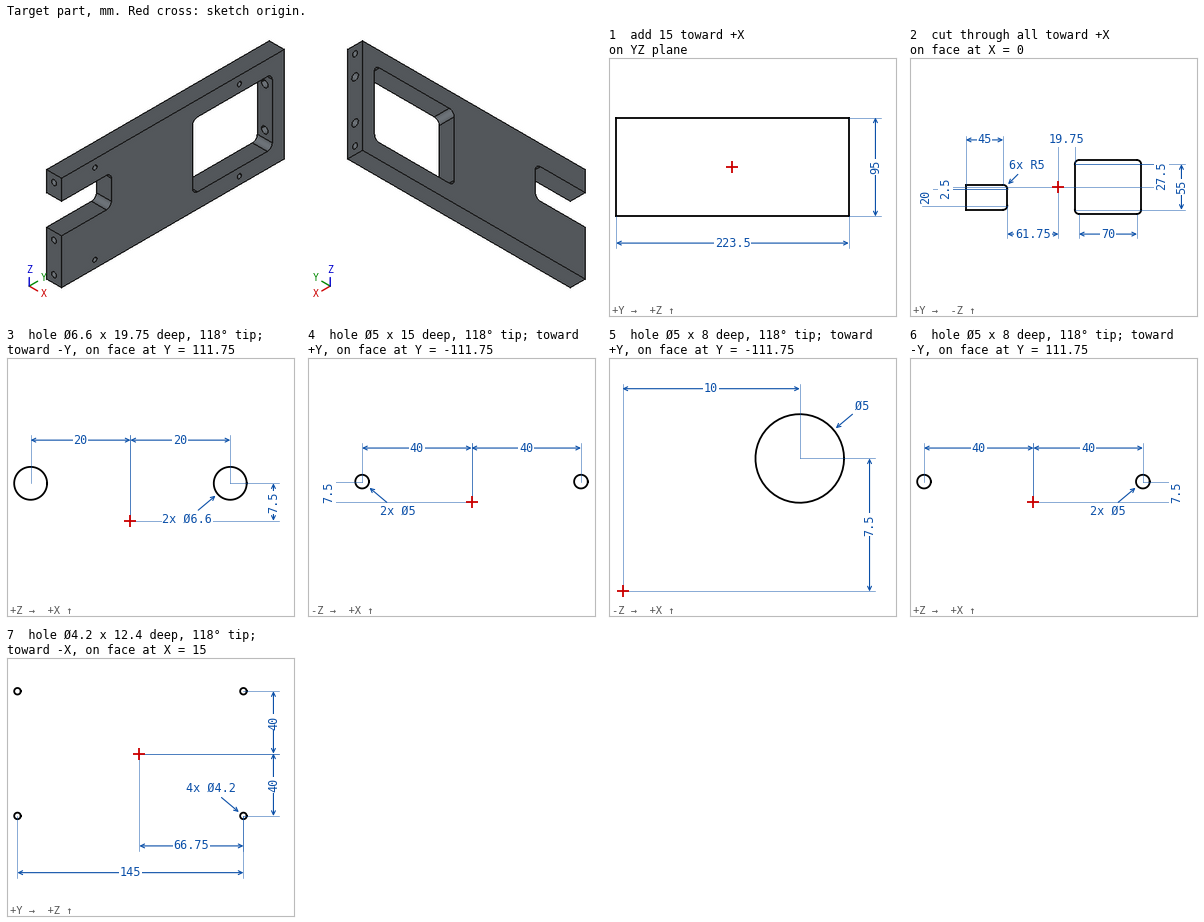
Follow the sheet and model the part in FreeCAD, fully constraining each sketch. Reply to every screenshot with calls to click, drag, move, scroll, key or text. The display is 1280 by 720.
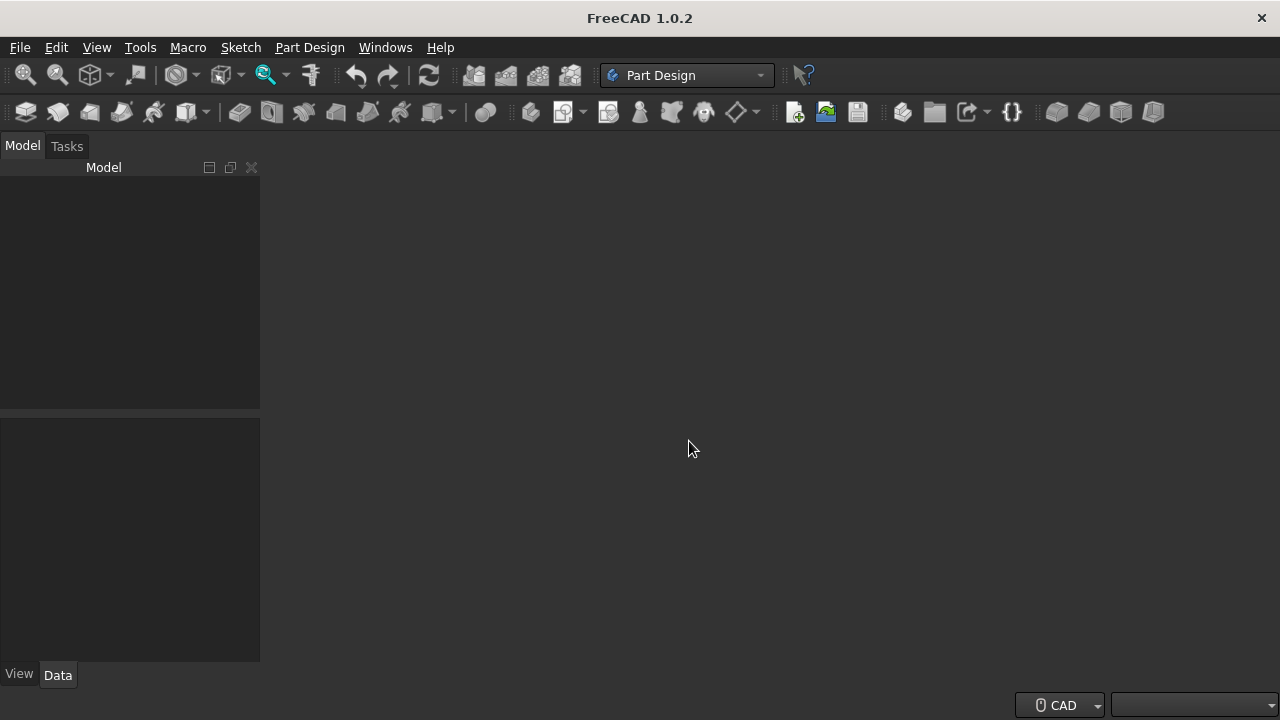
click(794, 112)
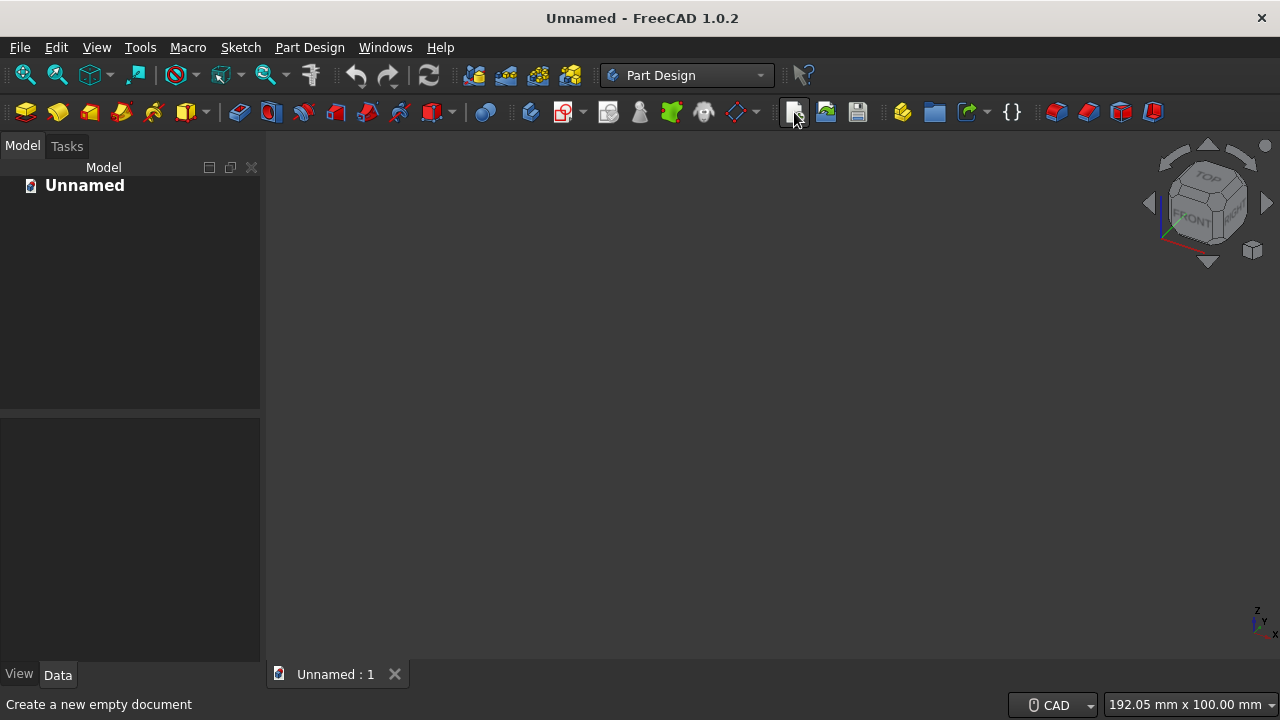
click(564, 112)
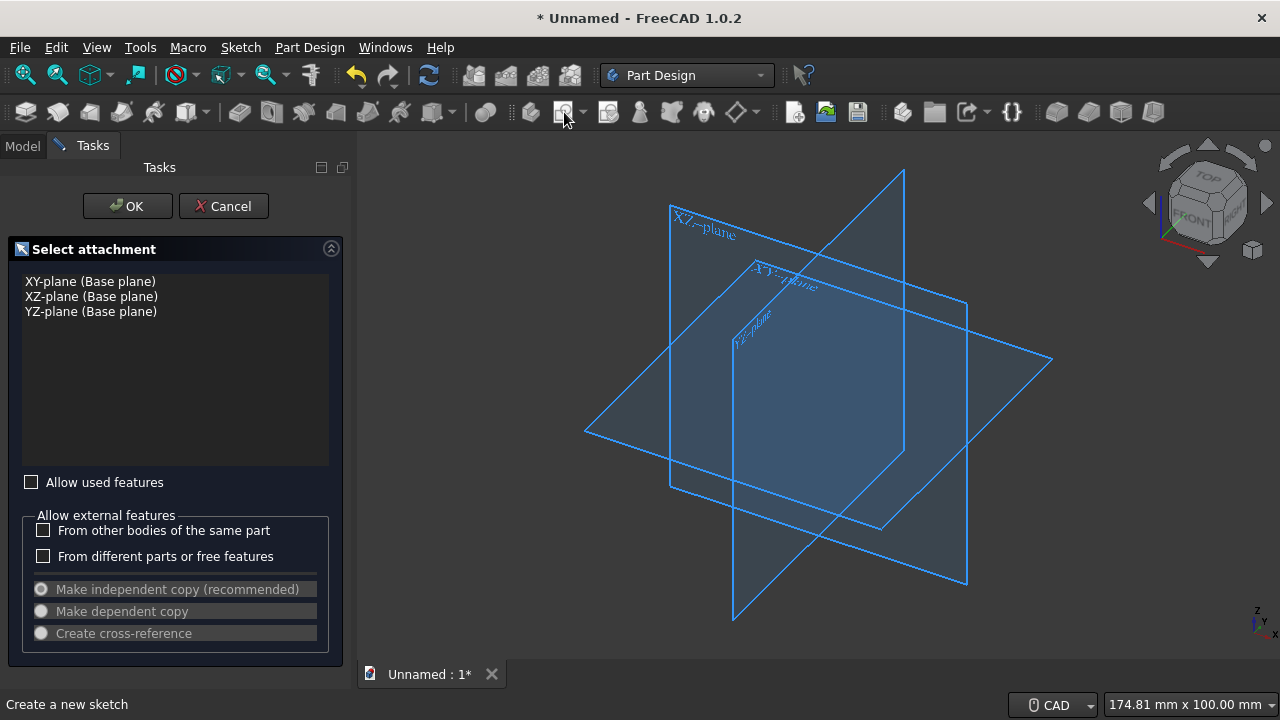
click(82, 312)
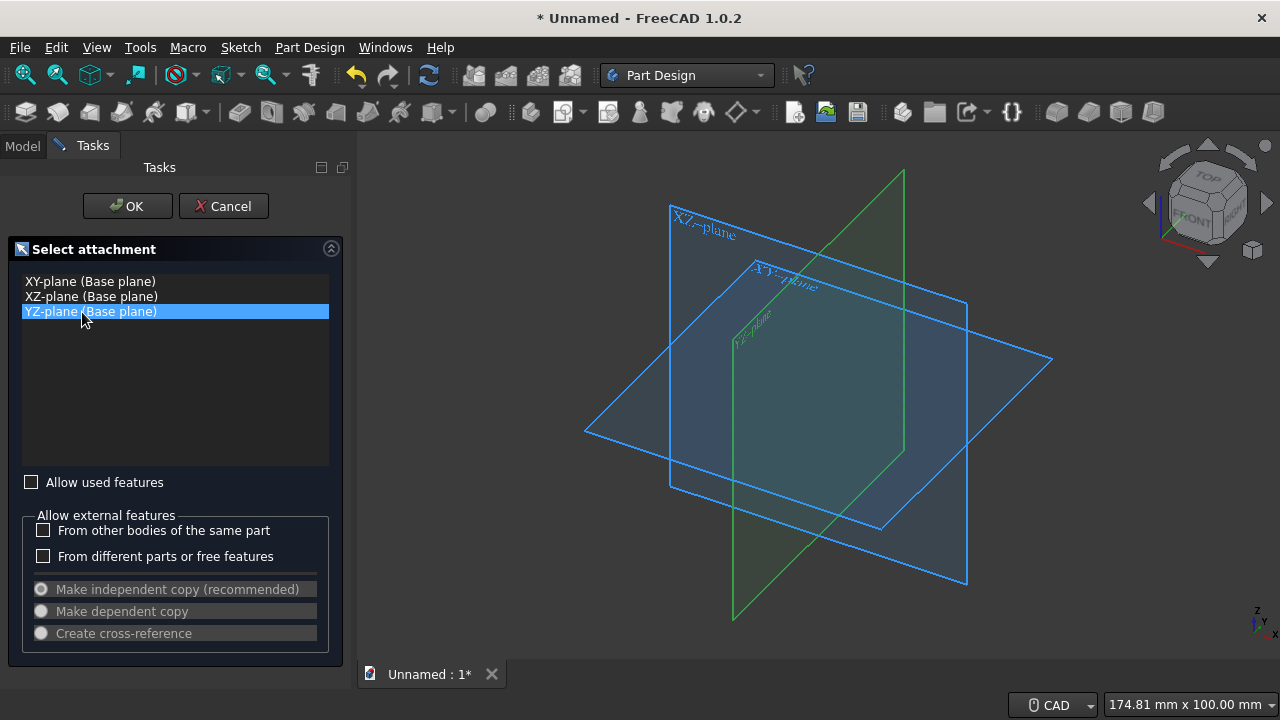
click(128, 206)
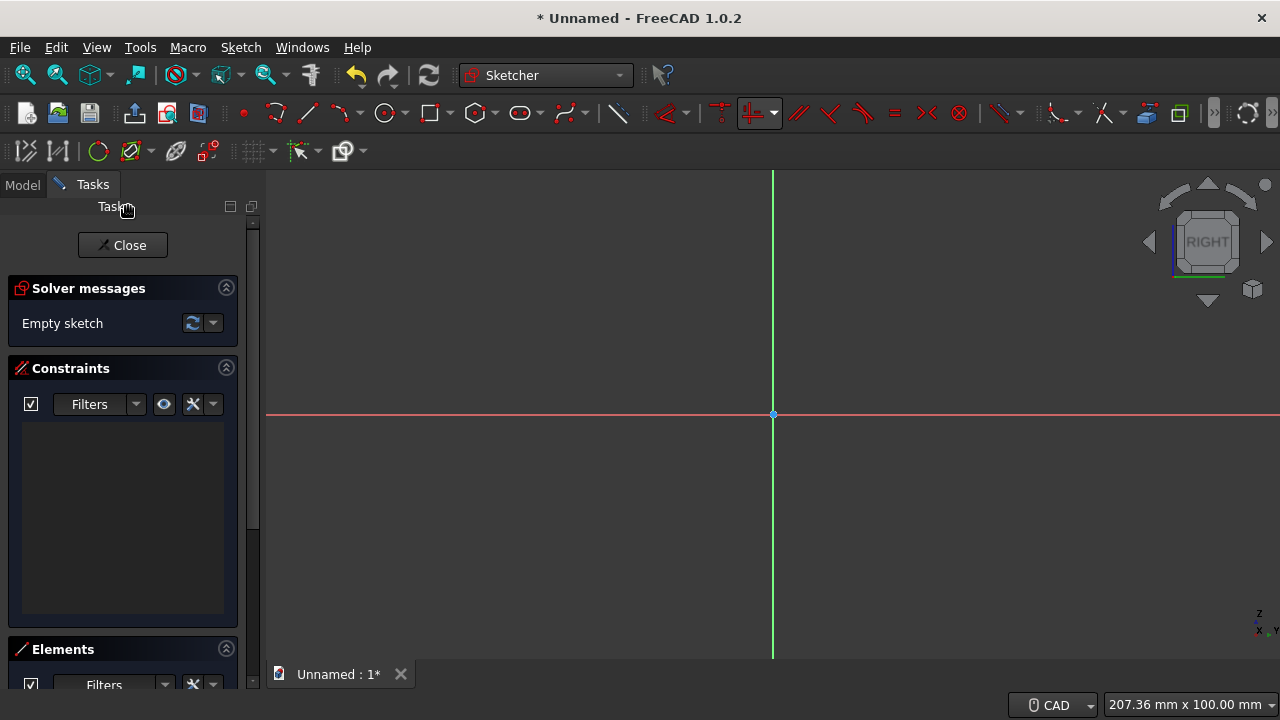
scroll(621, 414, down, 3)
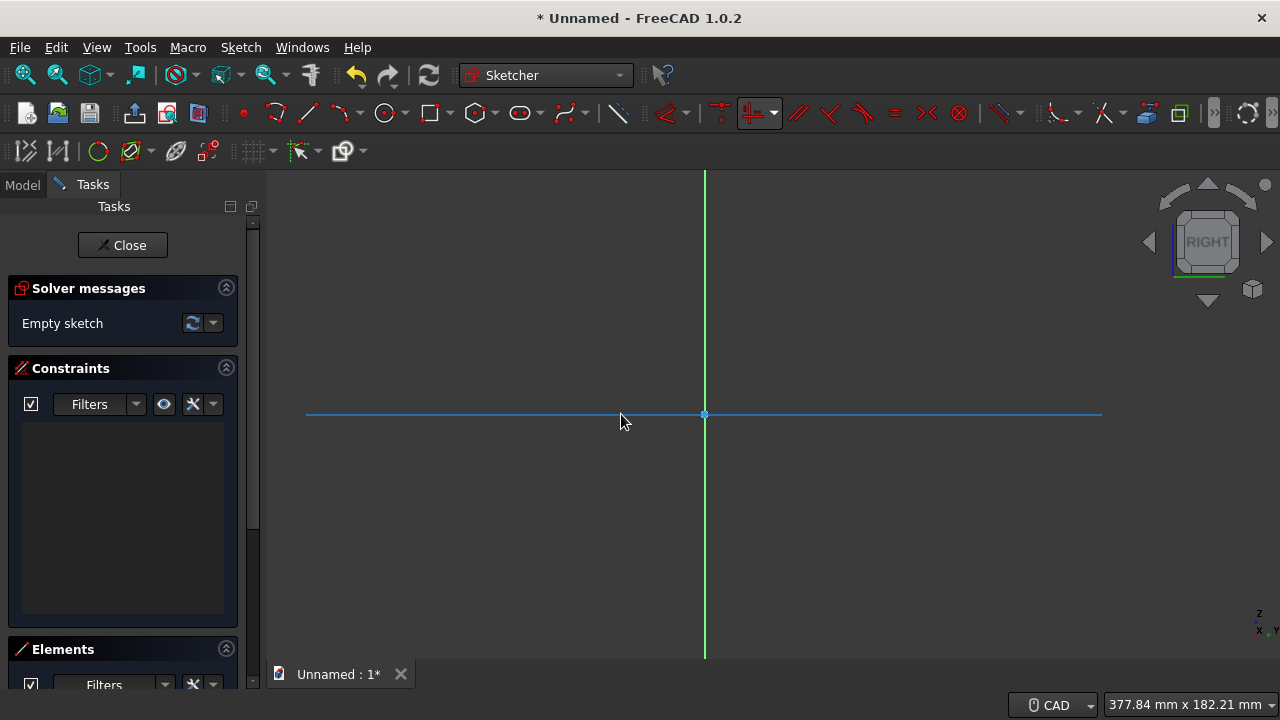
key(g)
key(v)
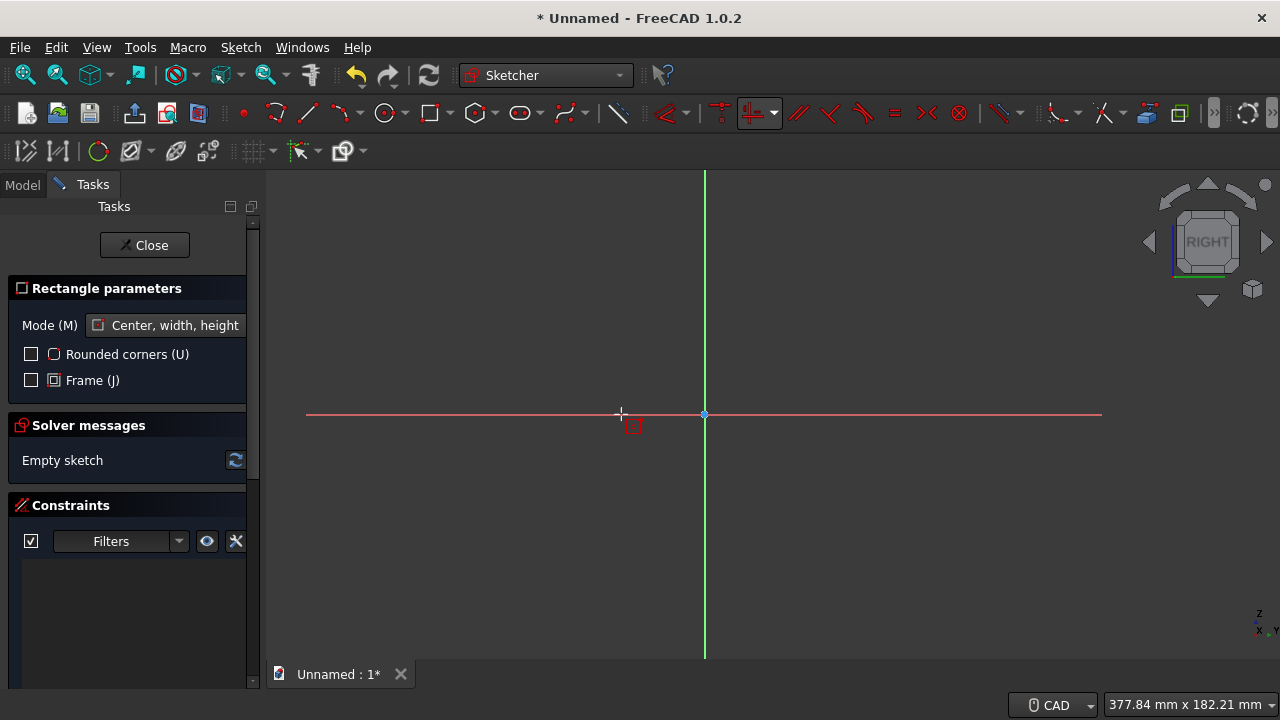
click(705, 414)
move(1004, 287)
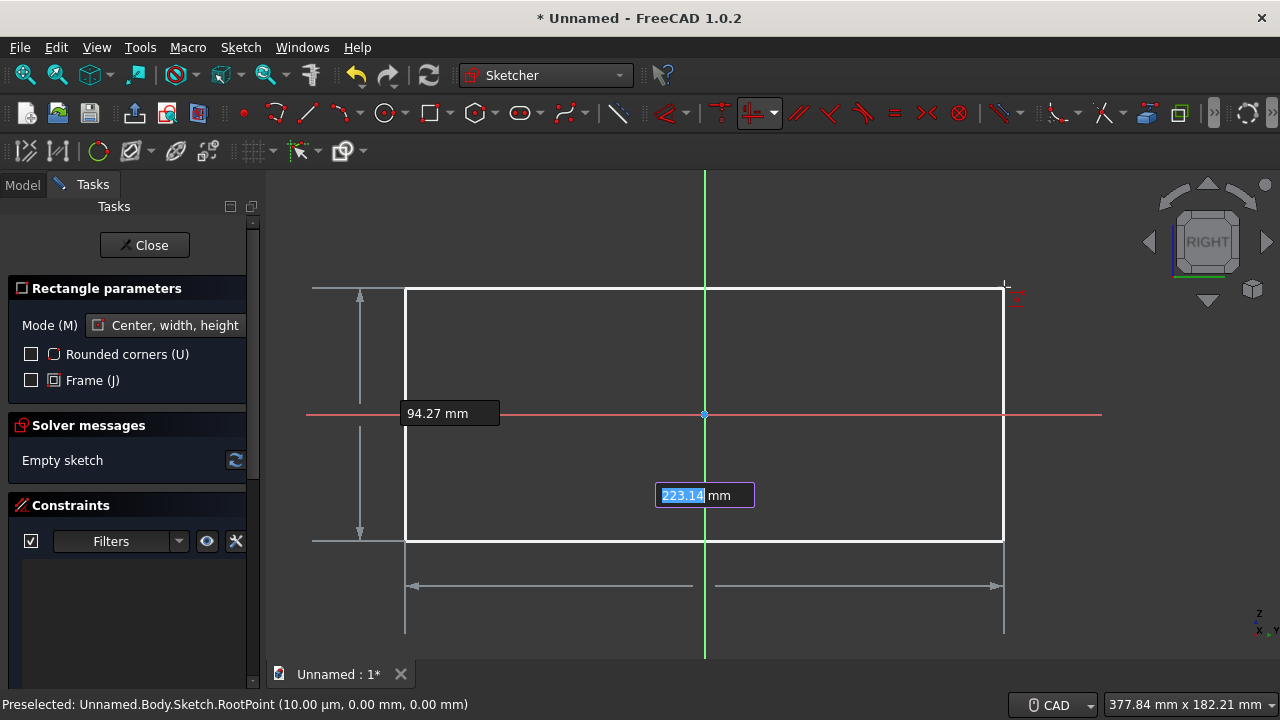
text(223.5)
key(Tab)
text(95)
key(Return)
key(Escape)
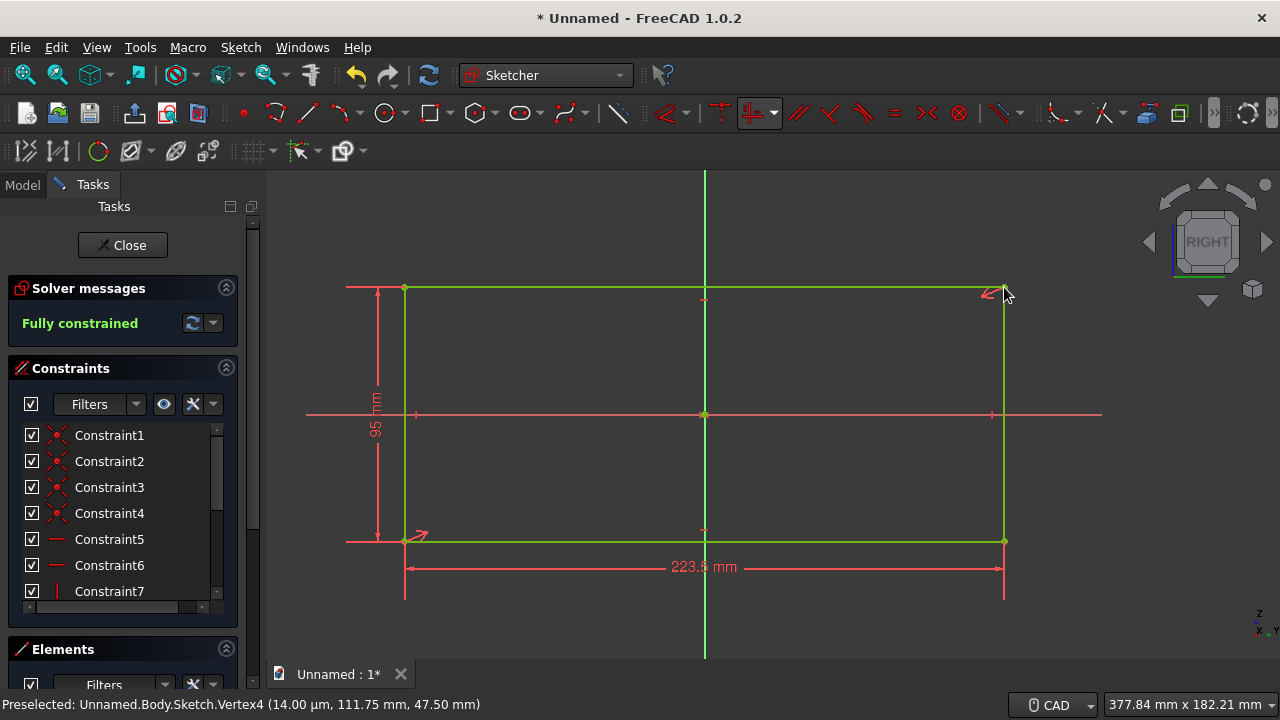
click(123, 245)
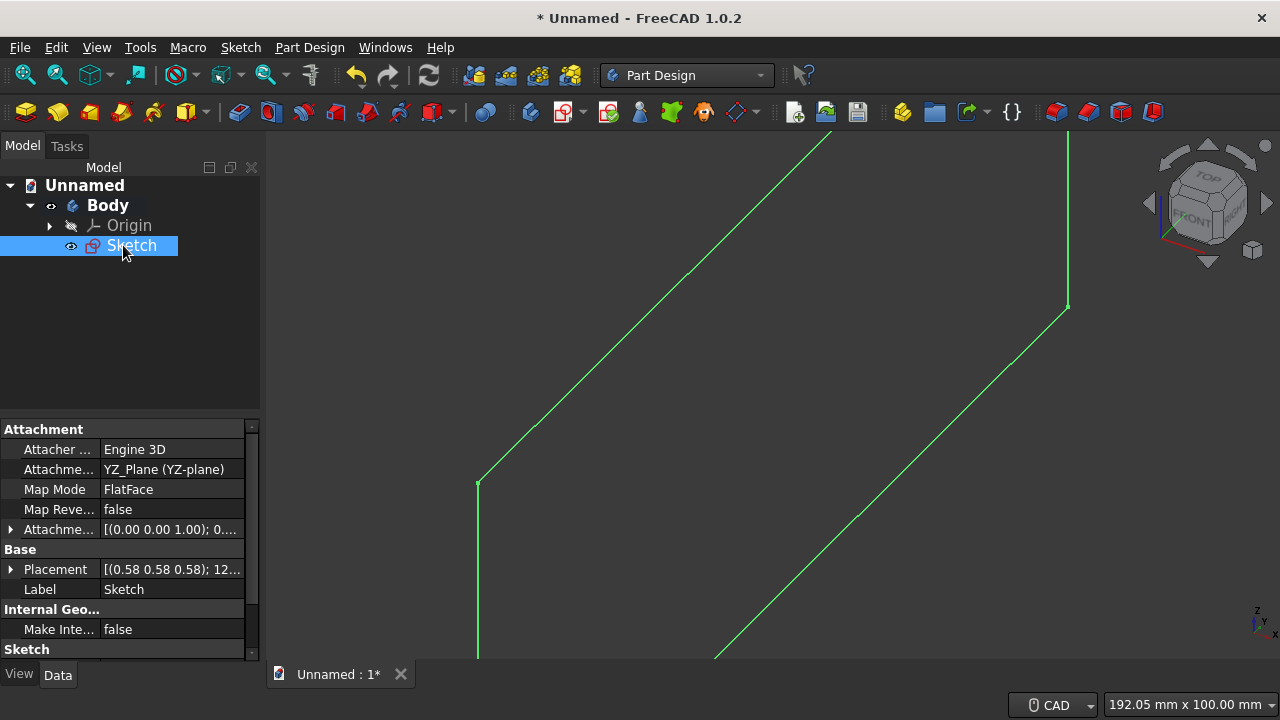
click(26, 112)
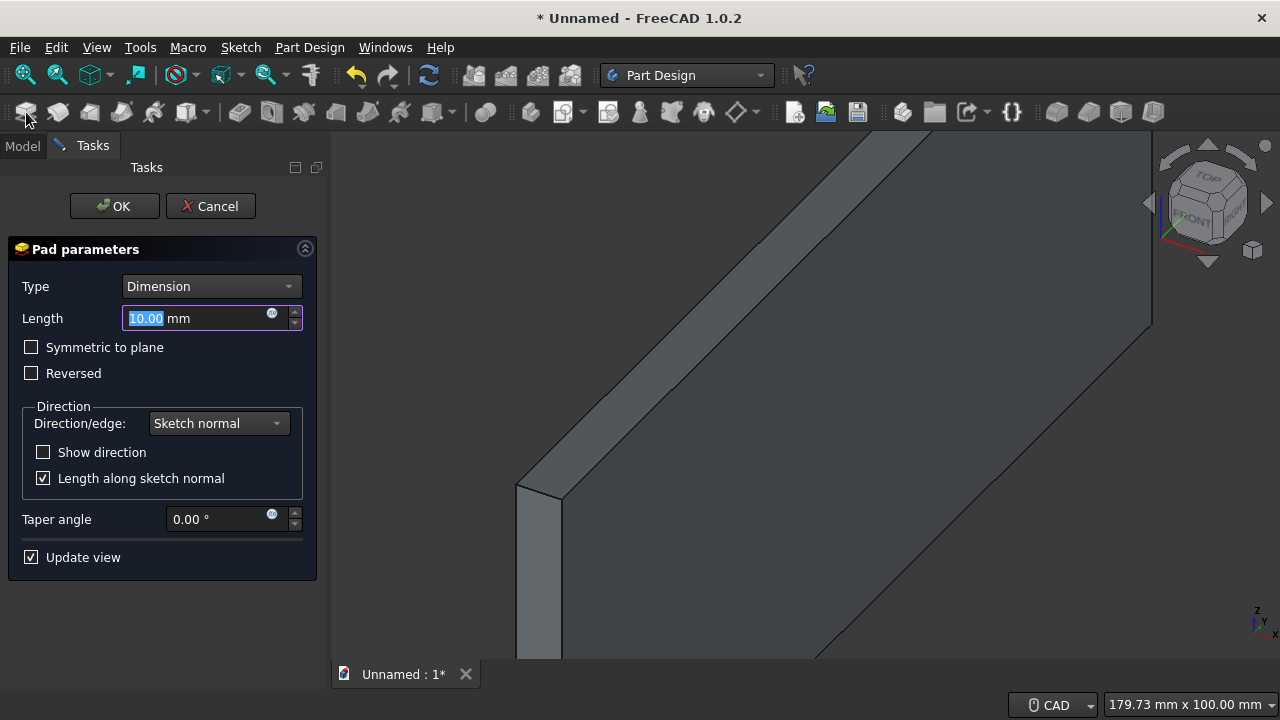
text(15)
key(Tab)